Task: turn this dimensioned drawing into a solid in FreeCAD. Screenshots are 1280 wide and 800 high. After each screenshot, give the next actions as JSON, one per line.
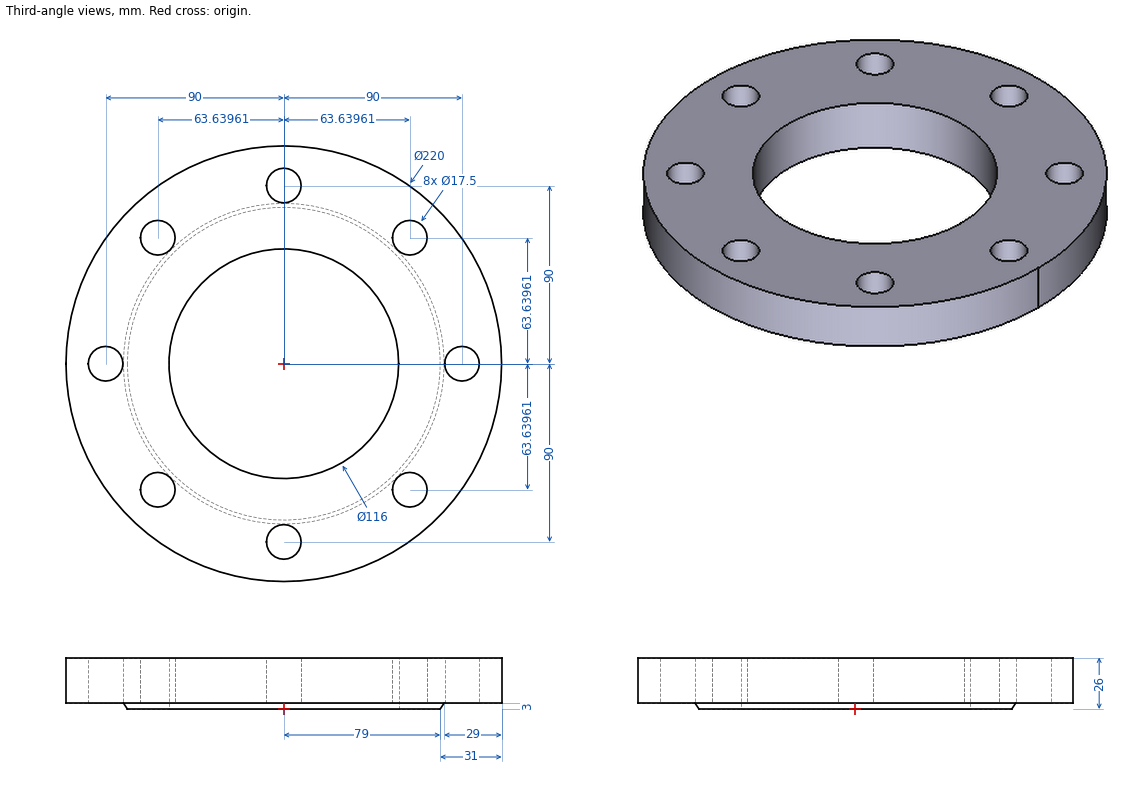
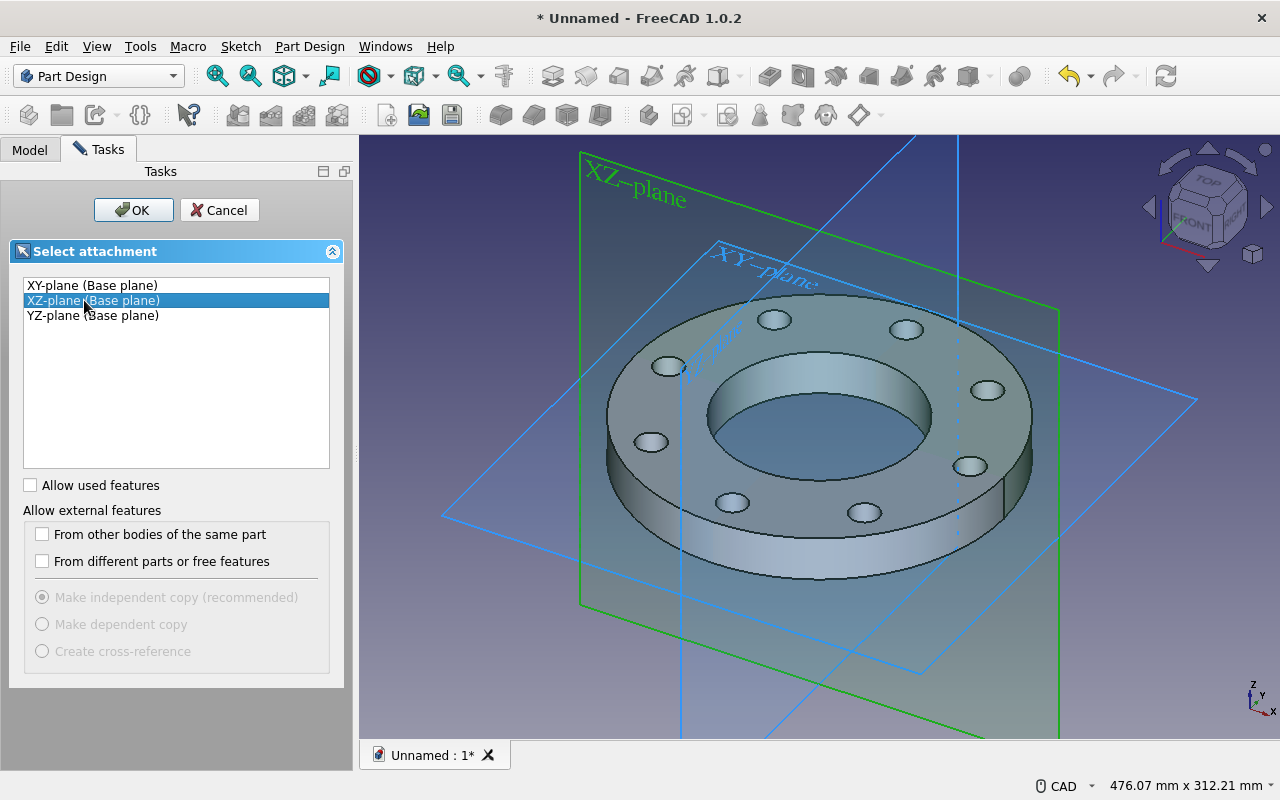
{"action": "left_click", "coordinate": [134, 210]}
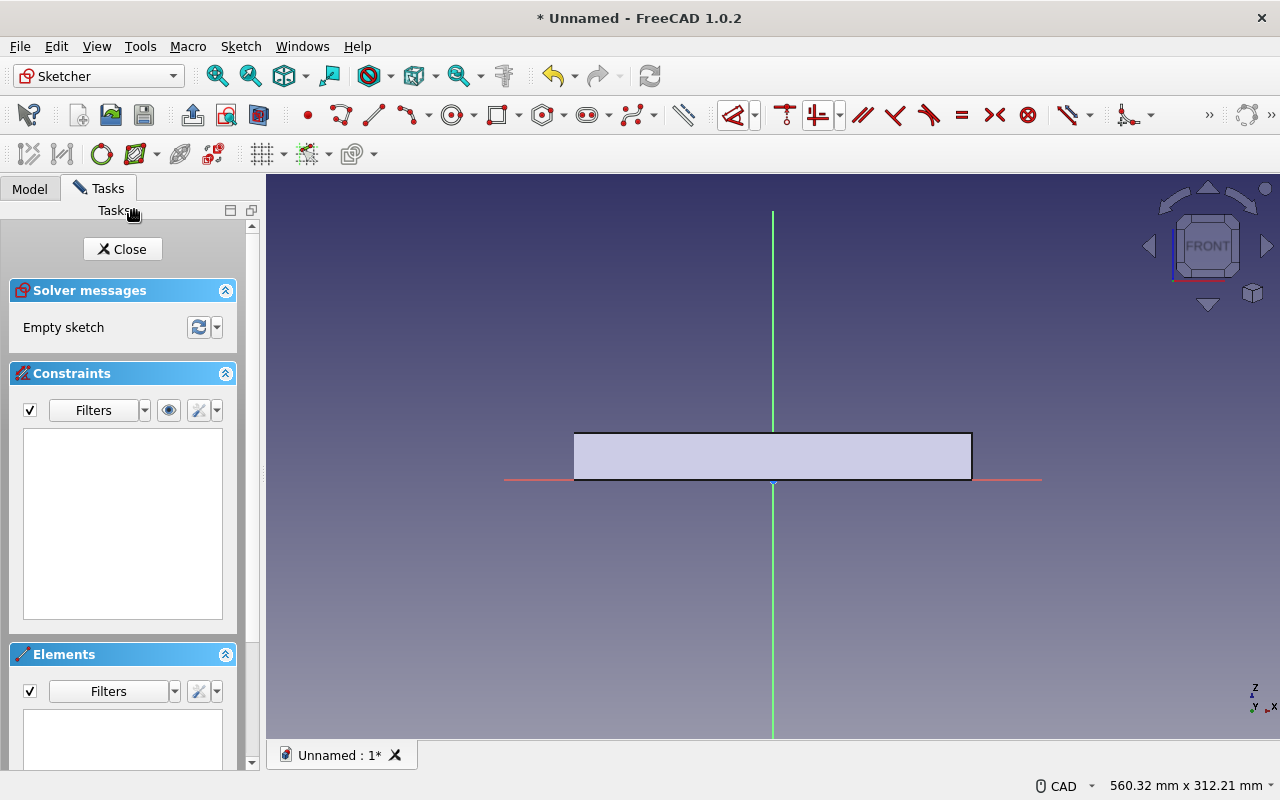
{"action": "key", "text": "q s"}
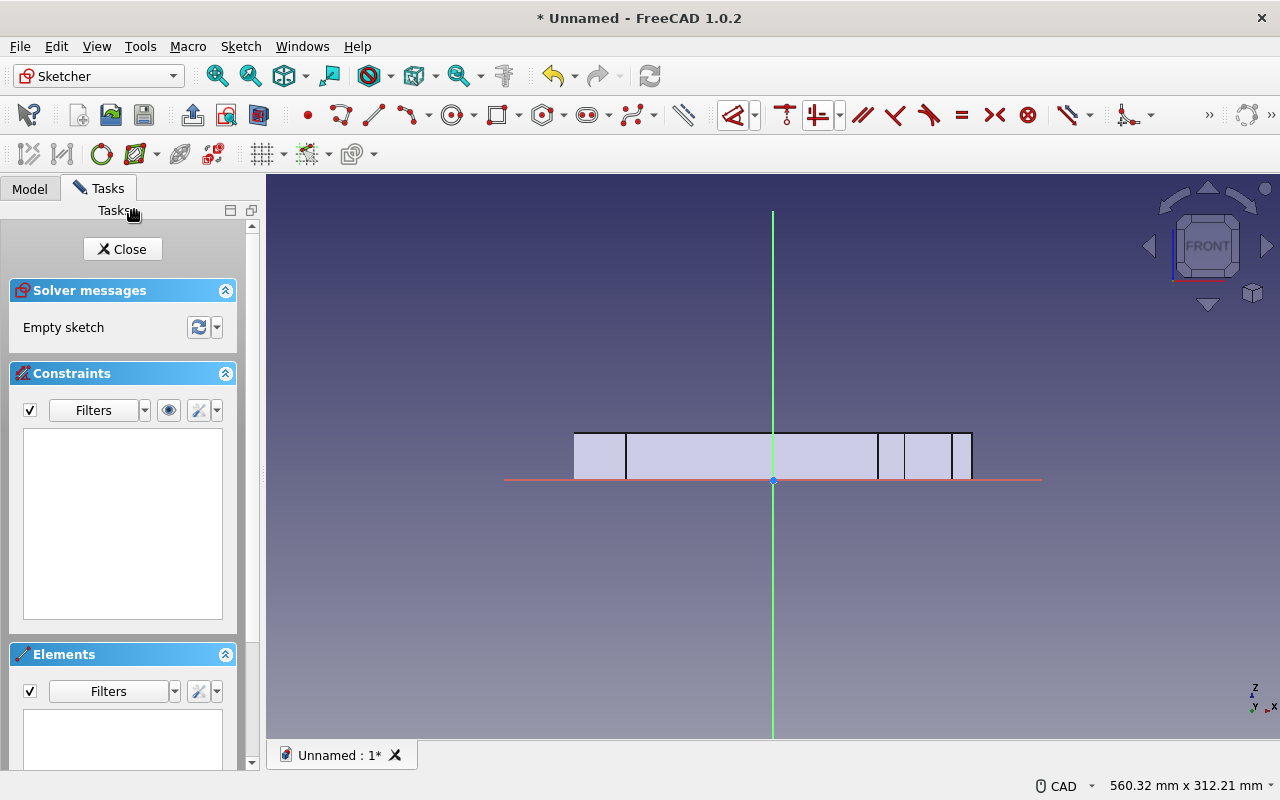
{"action": "scroll", "coordinate": [968, 479], "scroll_direction": "up", "scroll_amount": 12}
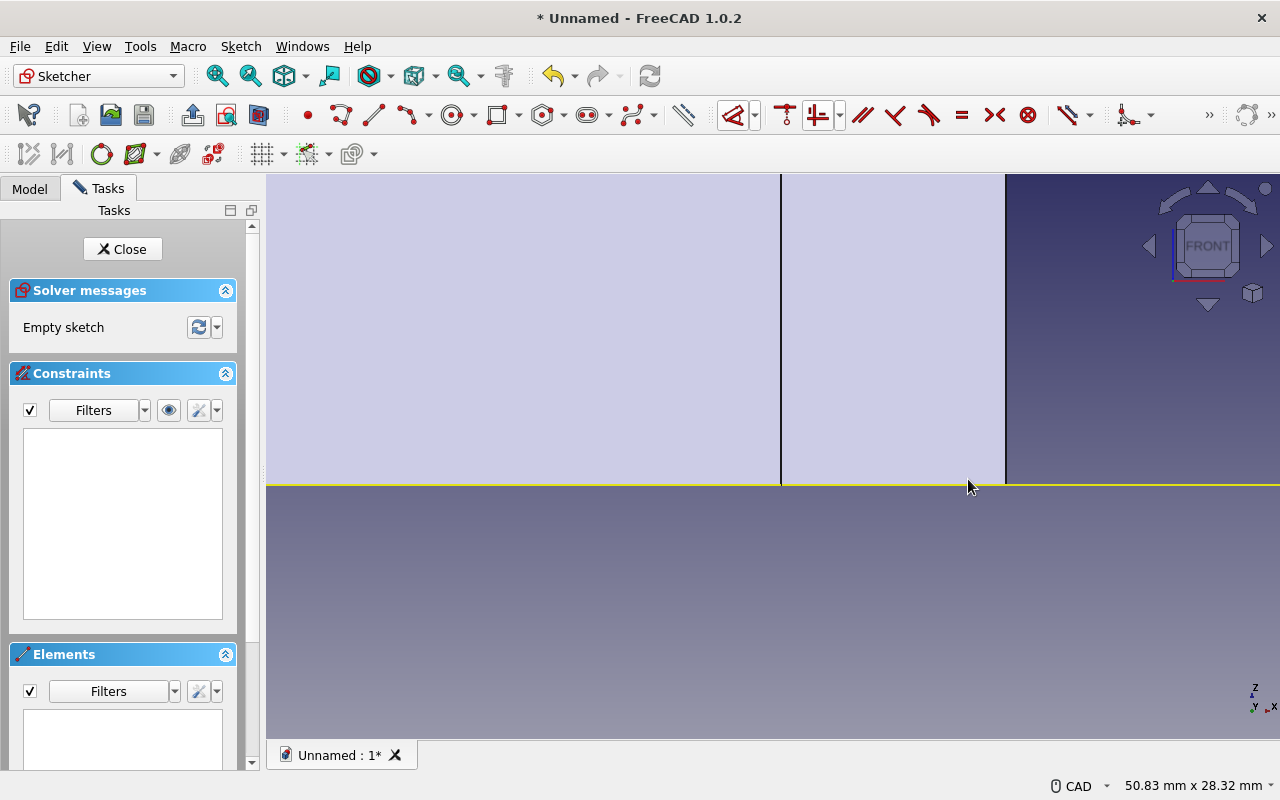
{"action": "left_click", "coordinate": [341, 116]}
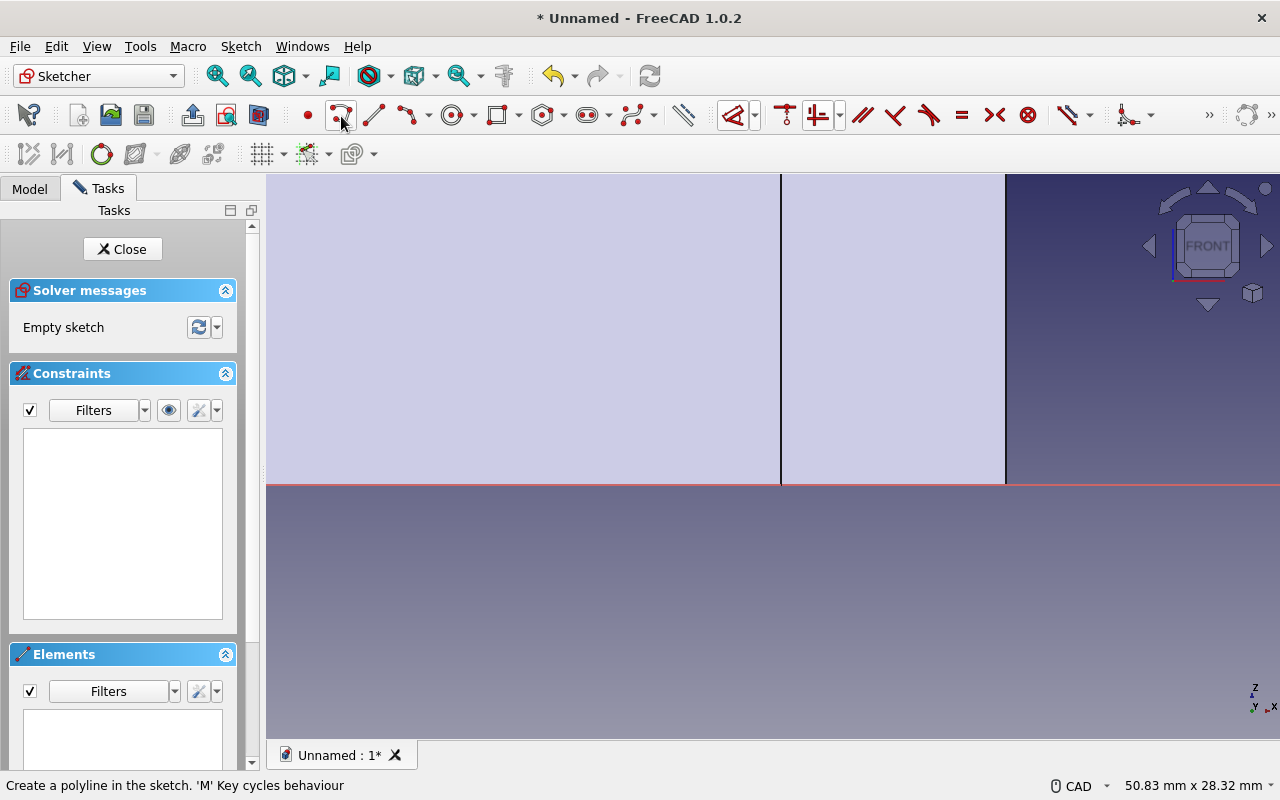
{"action": "left_click", "coordinate": [387, 485]}
{"action": "left_click", "coordinate": [427, 425]}
{"action": "left_click", "coordinate": [1006, 425]}
{"action": "left_click", "coordinate": [1006, 476]}
{"action": "left_click", "coordinate": [387, 485]}
{"action": "key", "text": "Escape"}
{"action": "key", "text": "Escape"}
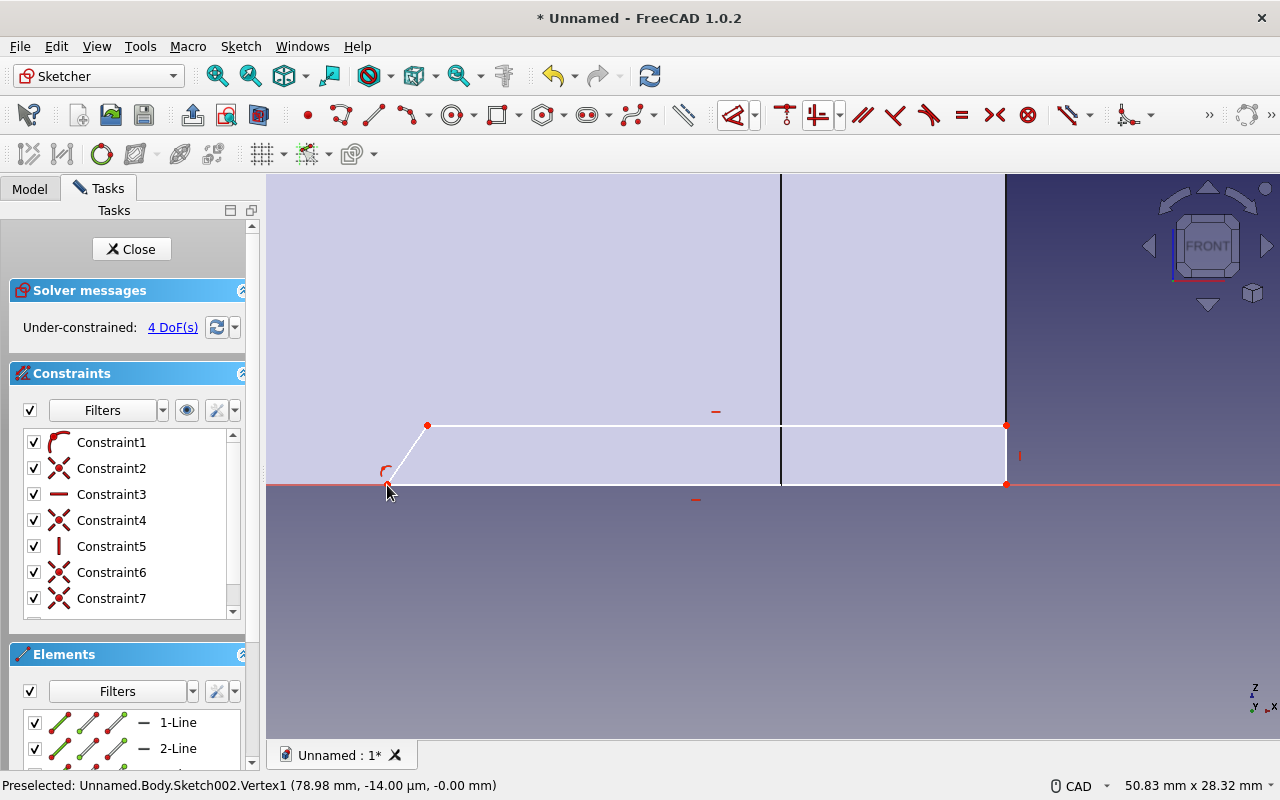
{"action": "left_click", "coordinate": [1006, 444]}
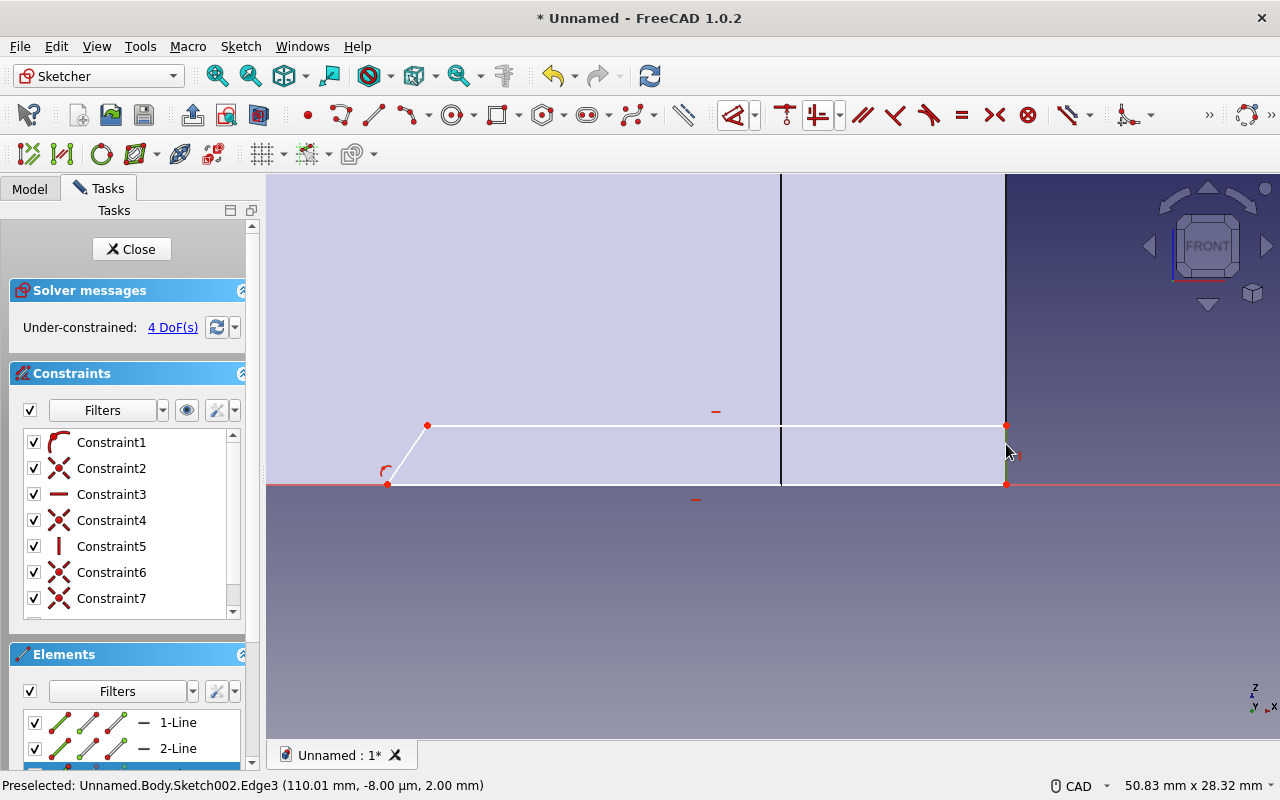
{"action": "left_click", "coordinate": [754, 116]}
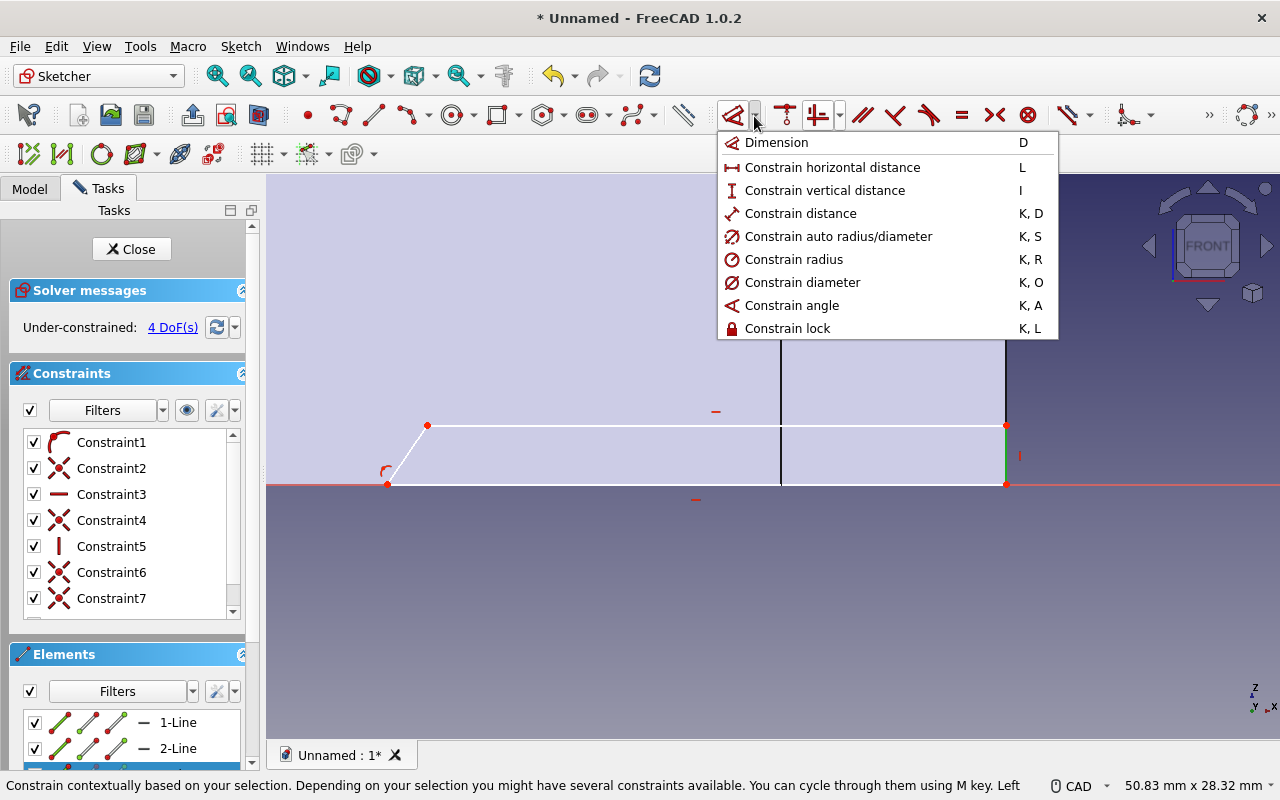
{"action": "left_click", "coordinate": [888, 190]}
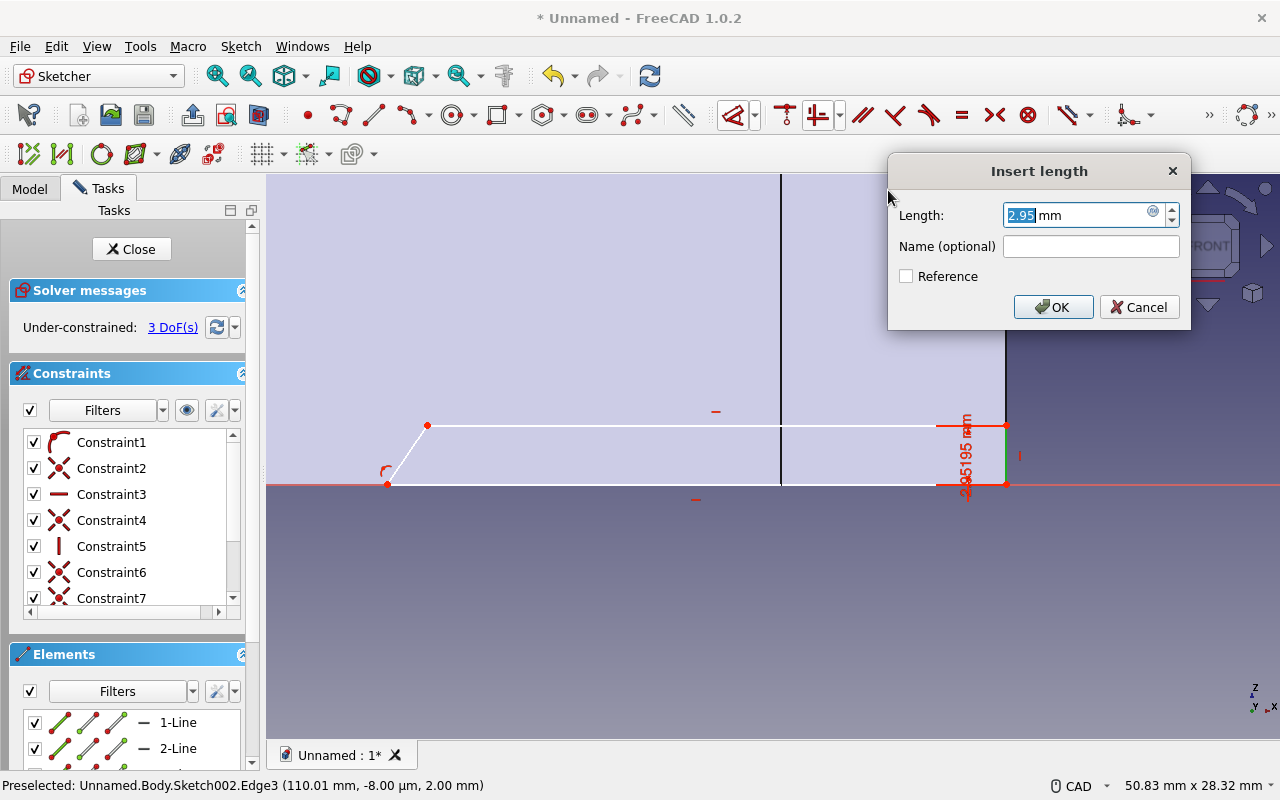
{"action": "type", "text": "3"}
{"action": "key", "text": "Return"}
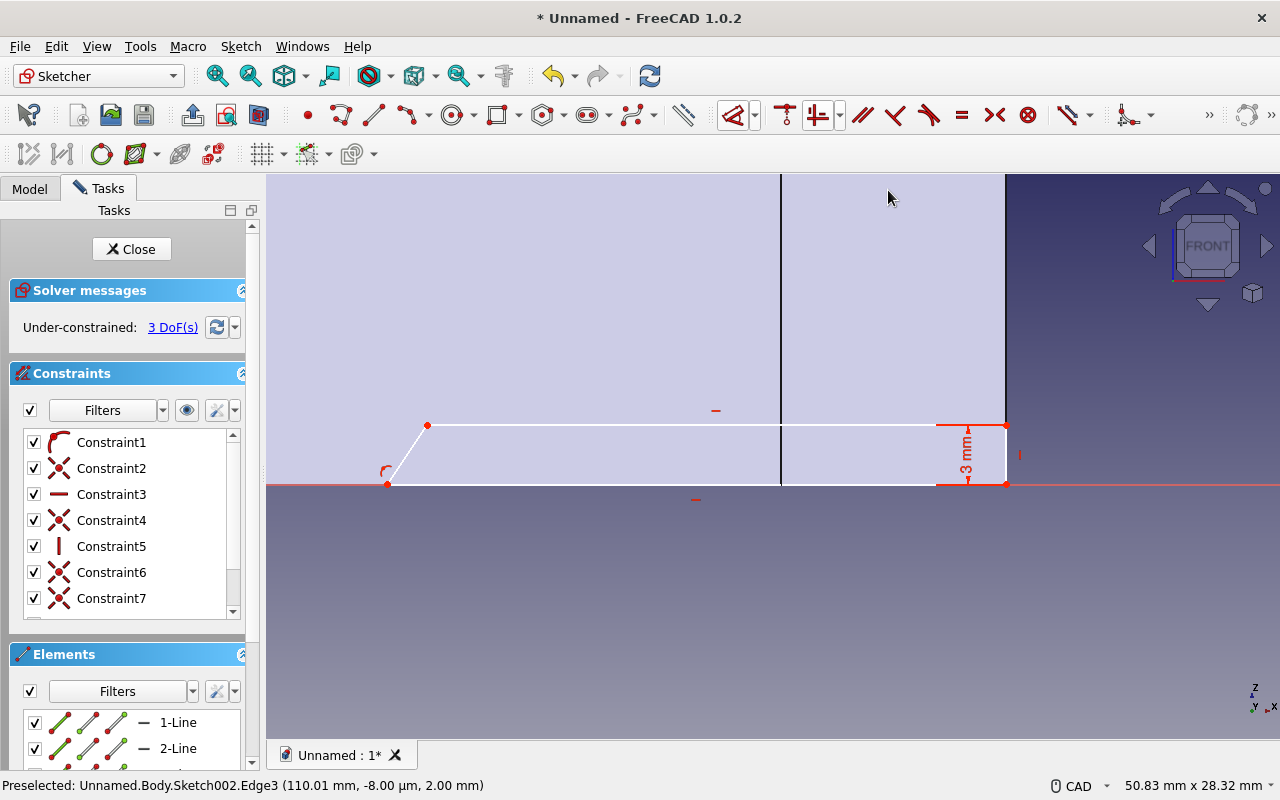
{"action": "left_click", "coordinate": [601, 425]}